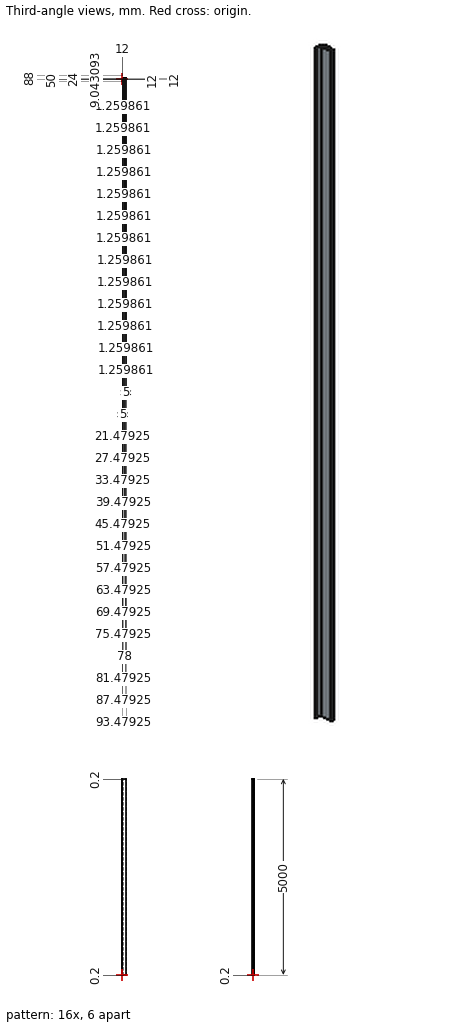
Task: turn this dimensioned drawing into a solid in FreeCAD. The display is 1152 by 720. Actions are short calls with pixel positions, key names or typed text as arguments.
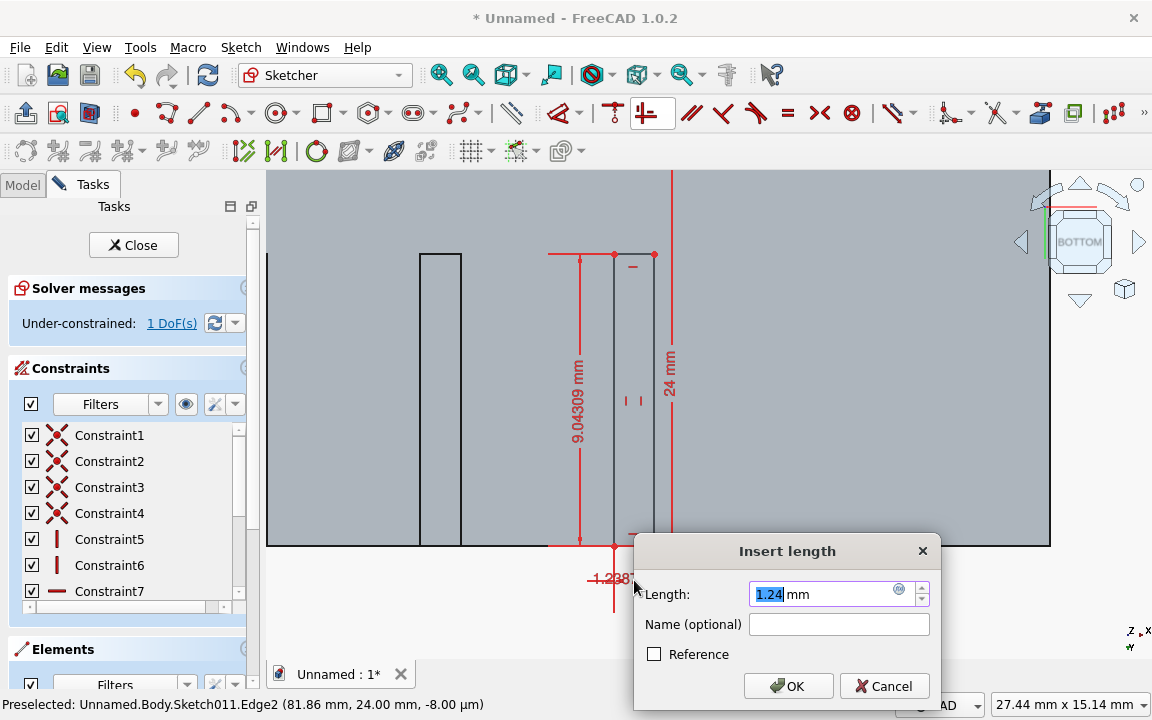
text(1.259861)
key(Return)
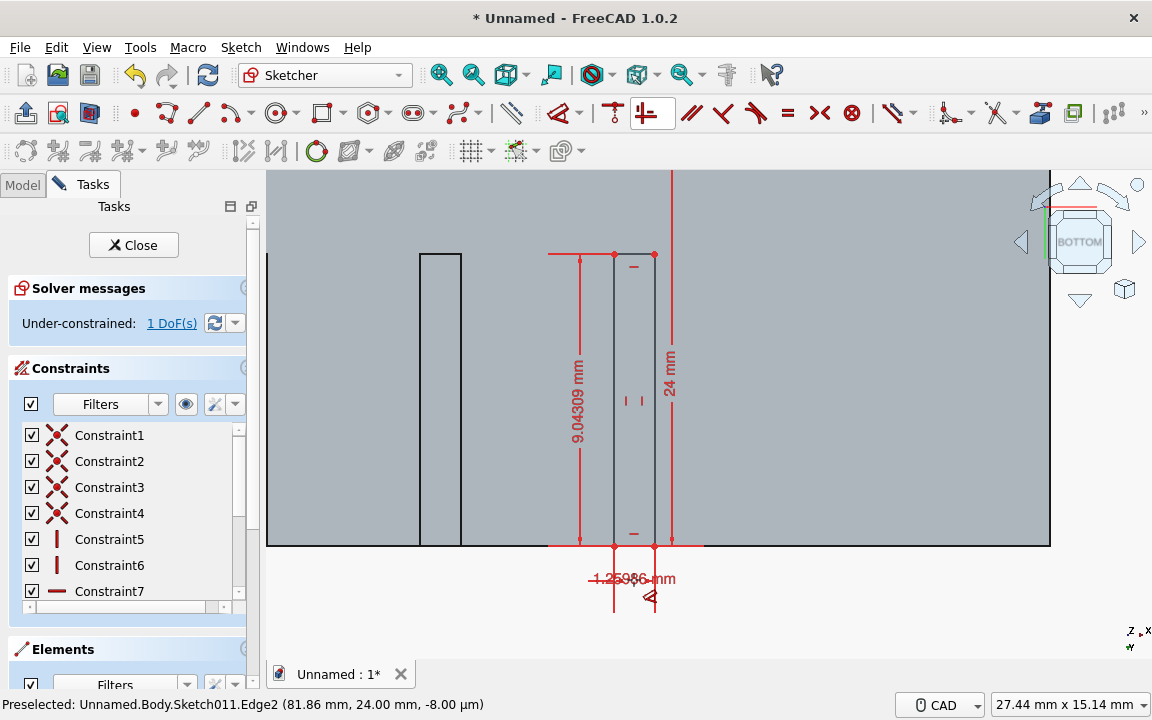
click(614, 254)
click(454, 288)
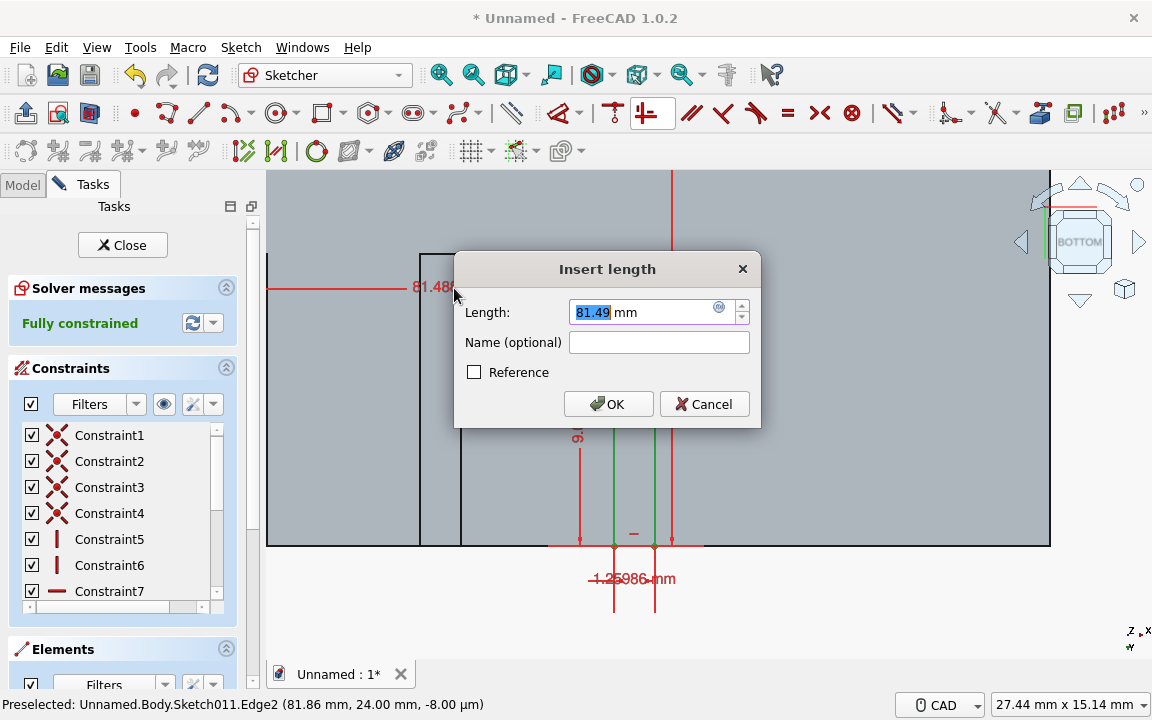
text(81.47925)
key(Return)
key(Escape)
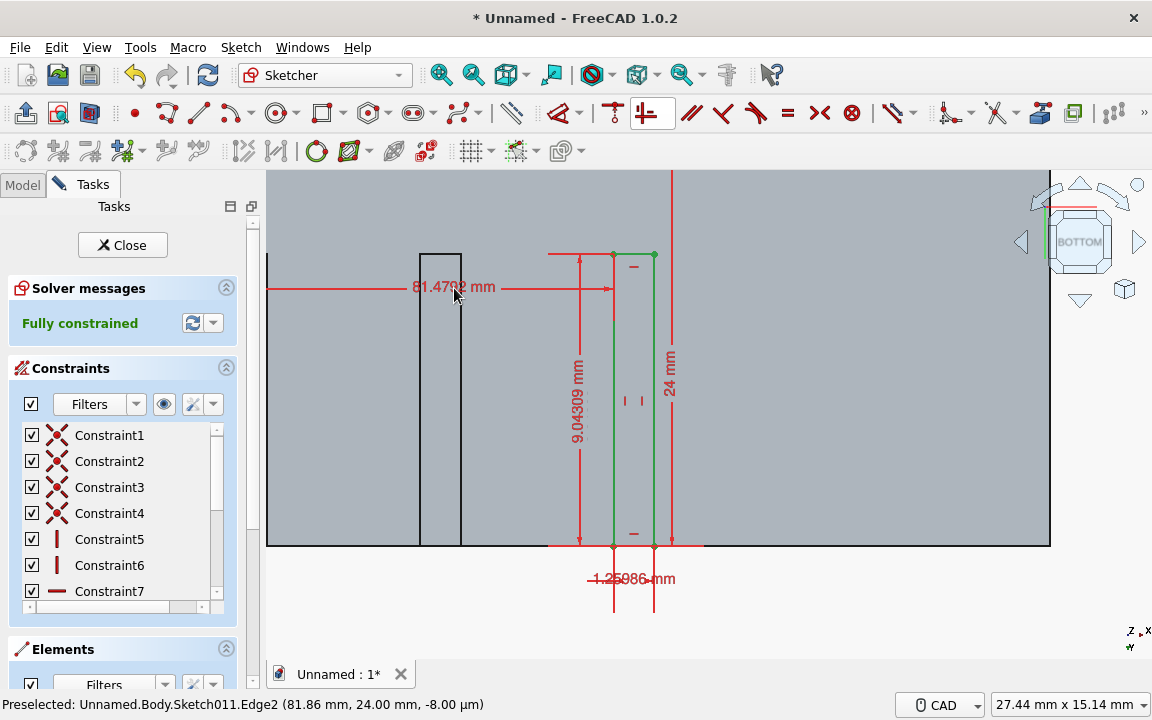
click(123, 245)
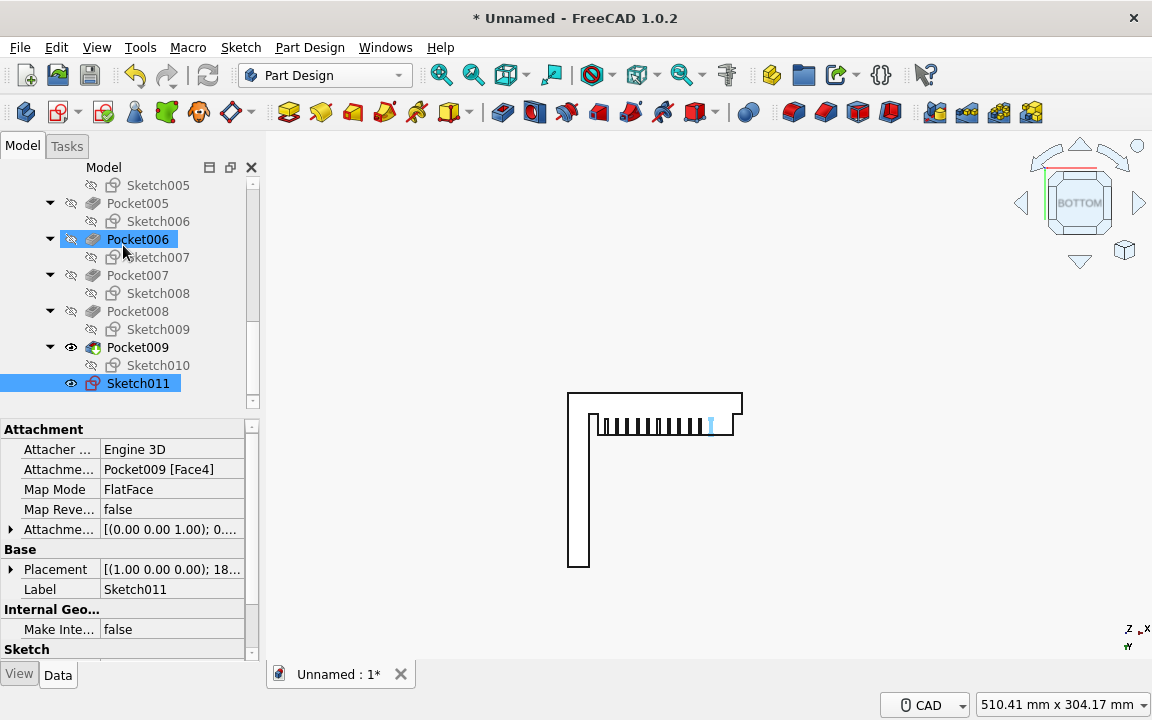
click(504, 112)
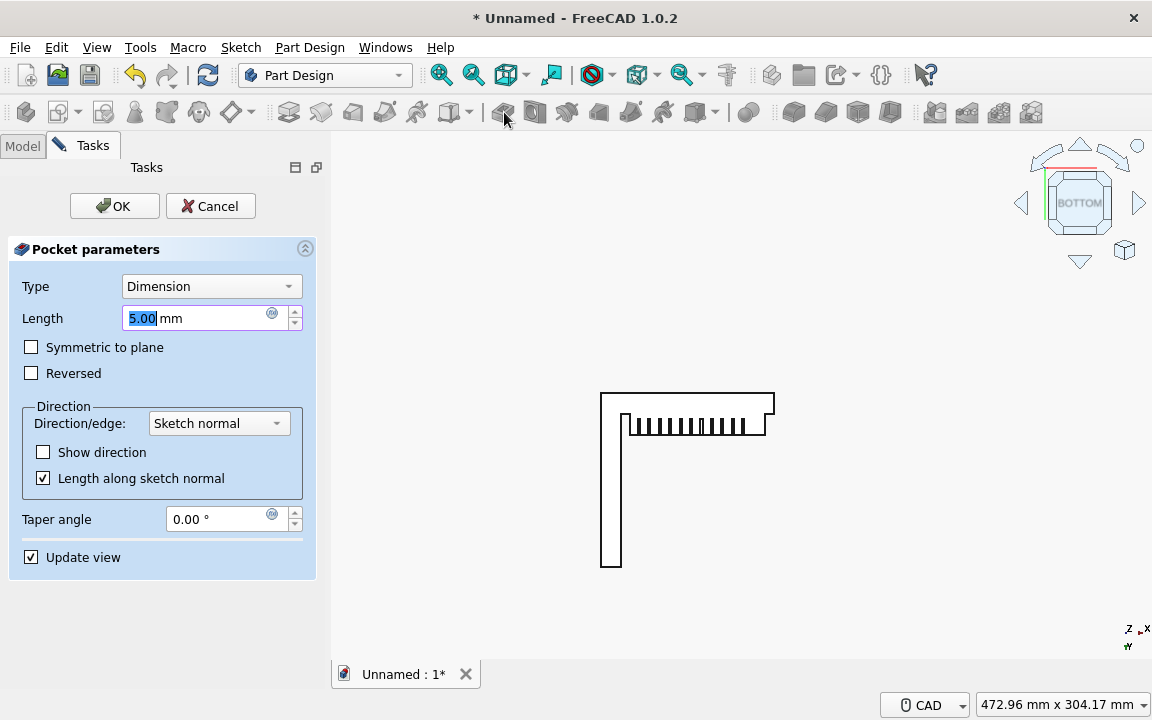
text(0.2)
key(Tab)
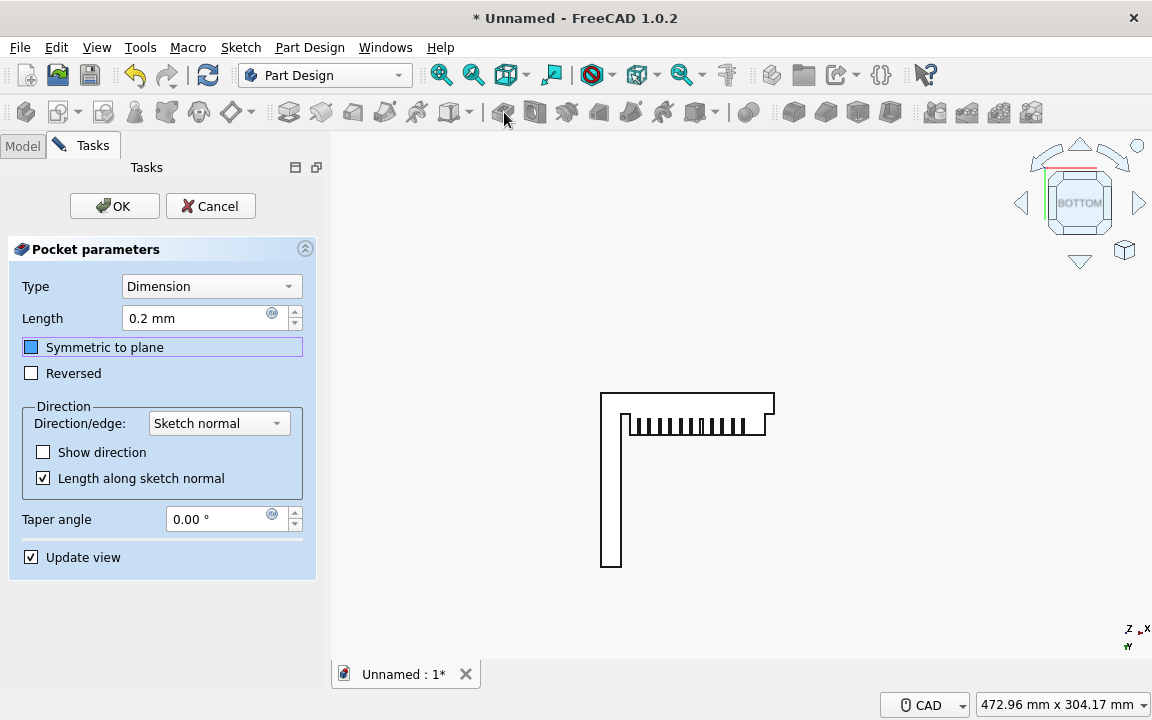
click(115, 206)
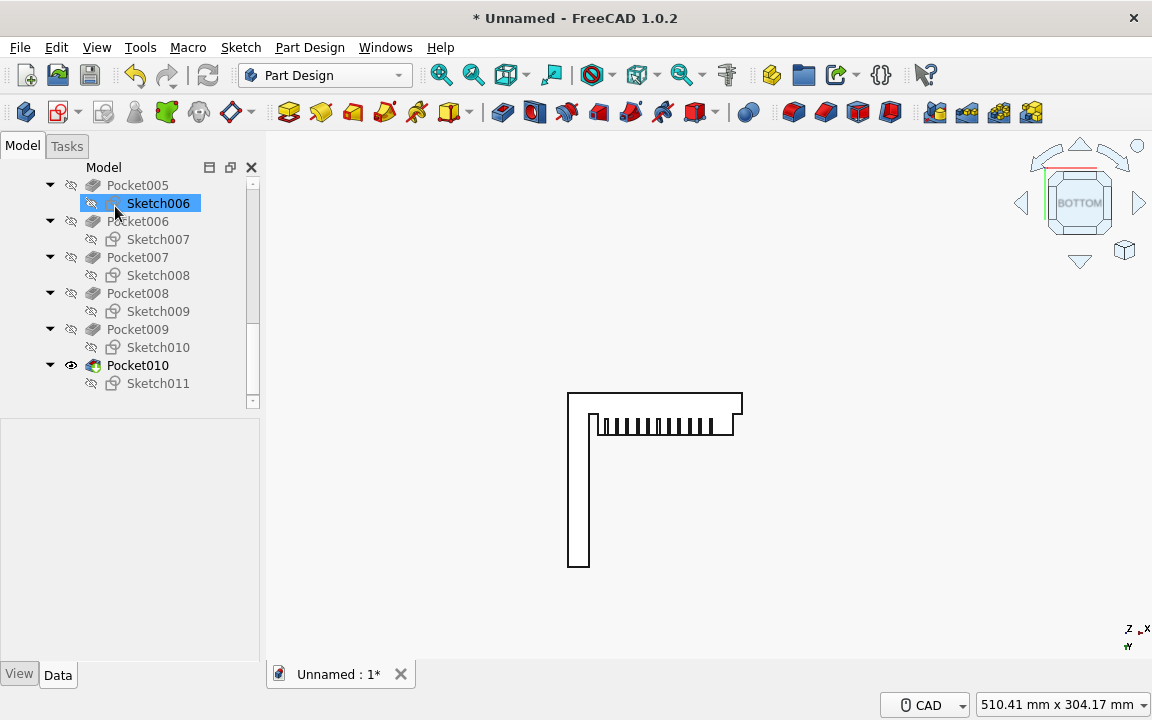
click(442, 76)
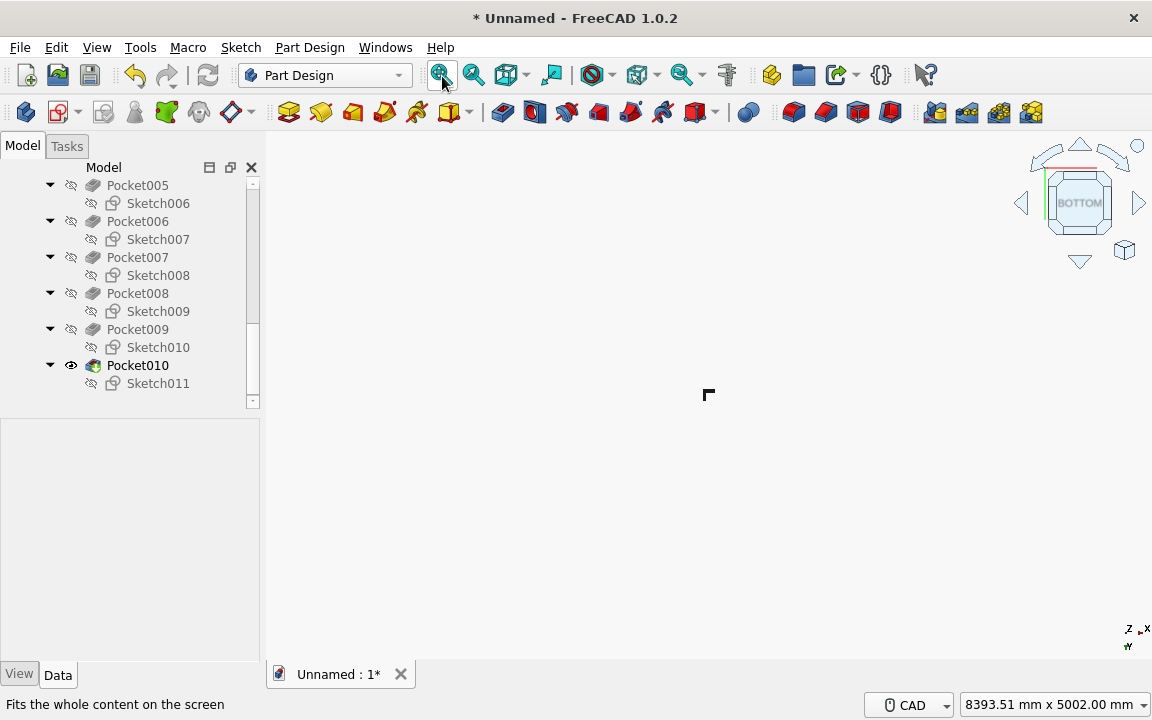
click(58, 112)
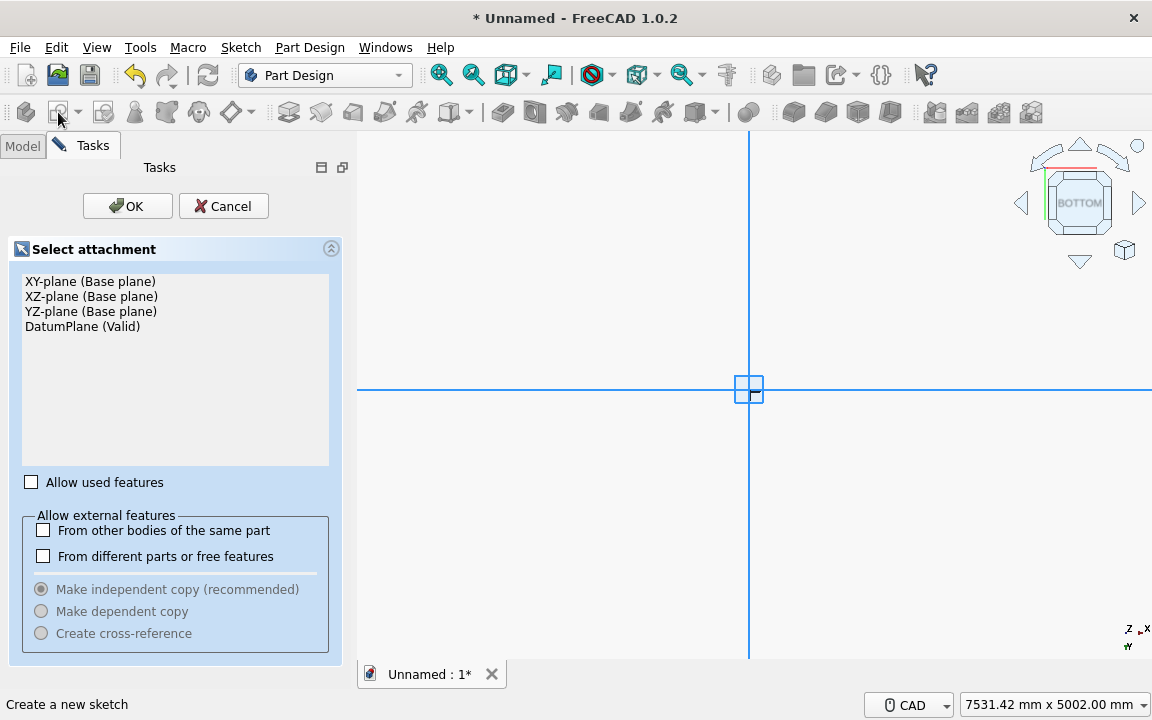
click(82, 282)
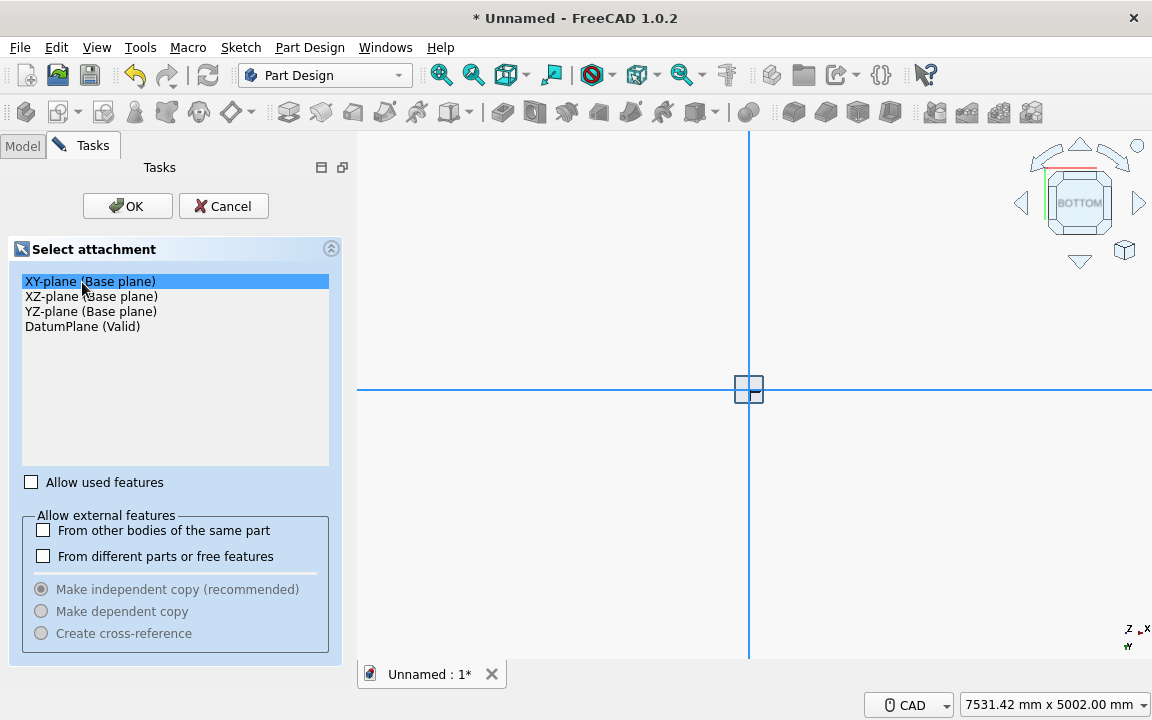
click(128, 206)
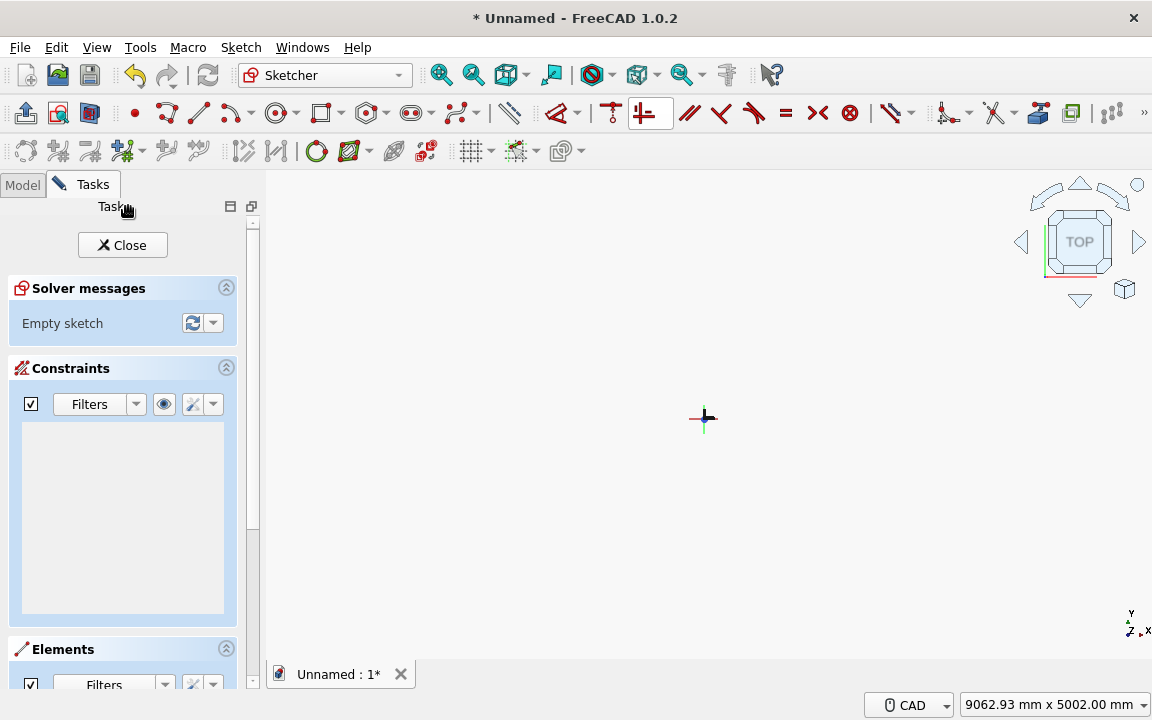
click(90, 114)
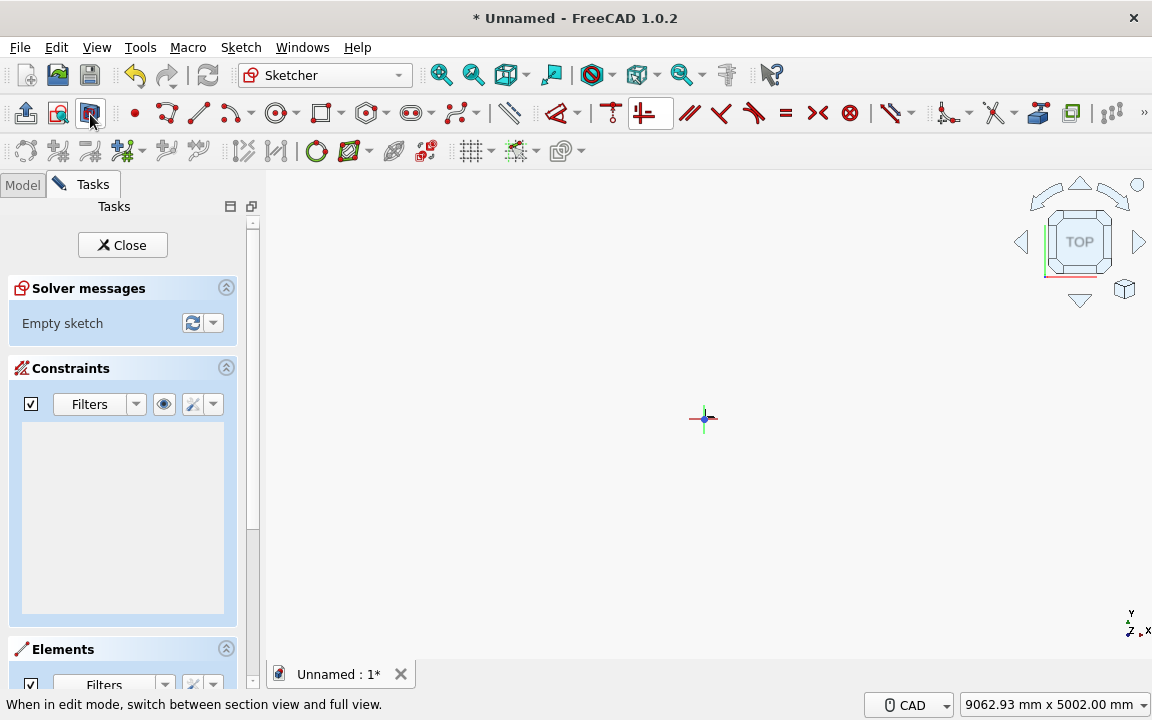
scroll(717, 418, up, 15)